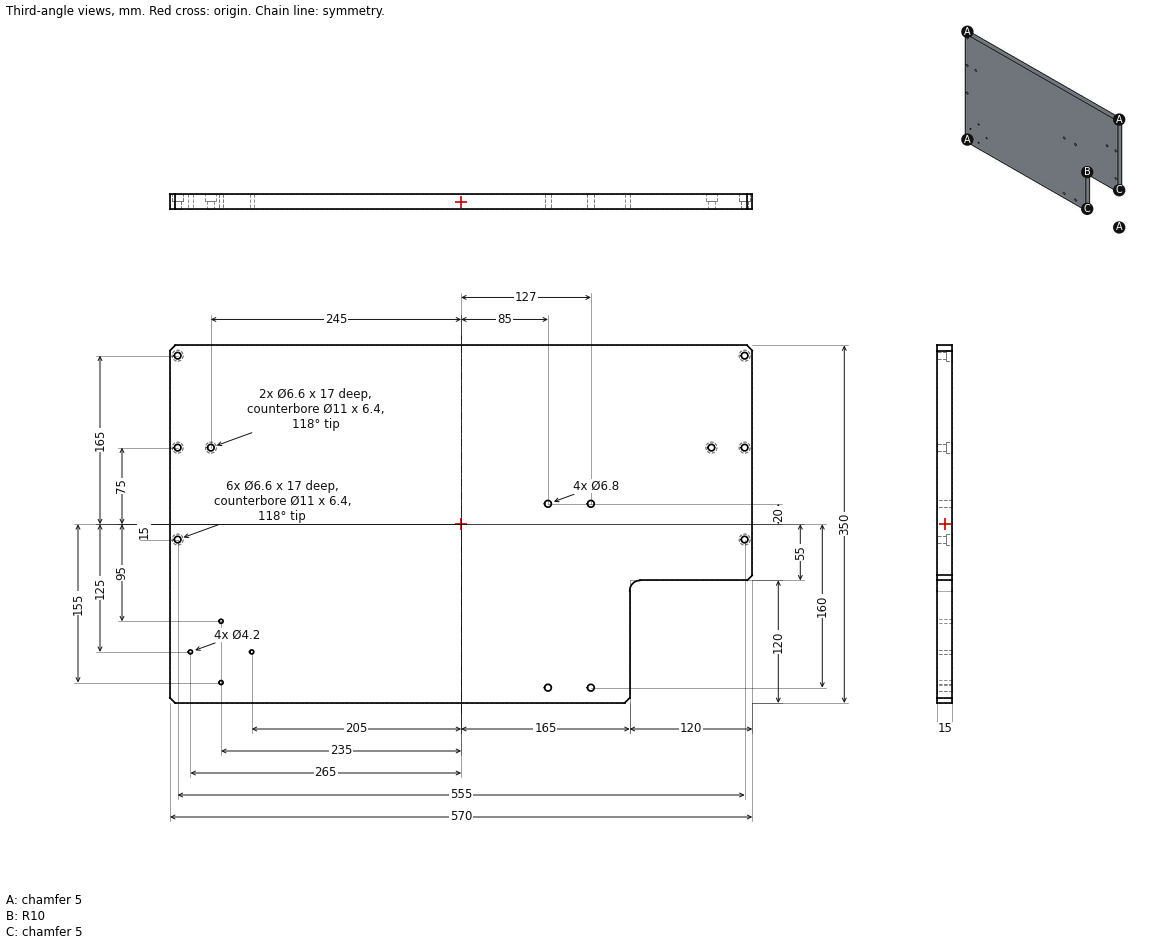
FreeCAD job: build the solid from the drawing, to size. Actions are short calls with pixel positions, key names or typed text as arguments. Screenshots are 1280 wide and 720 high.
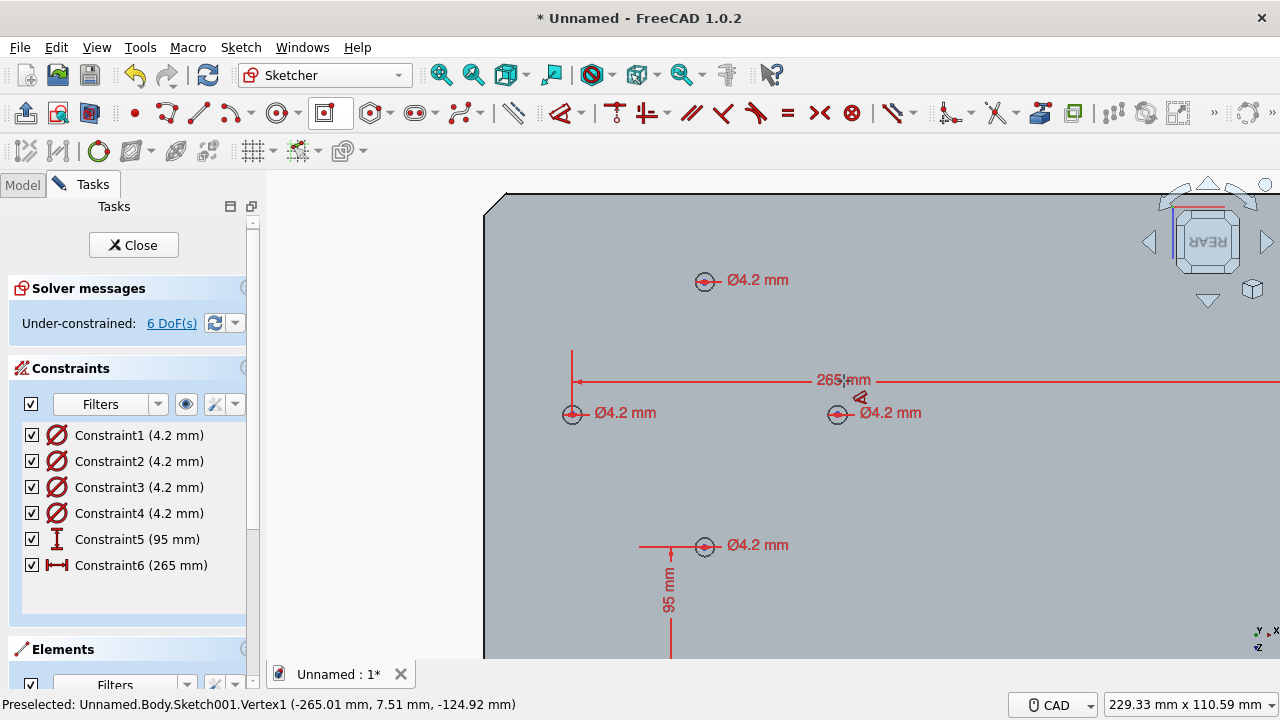
click(572, 415)
click(538, 523)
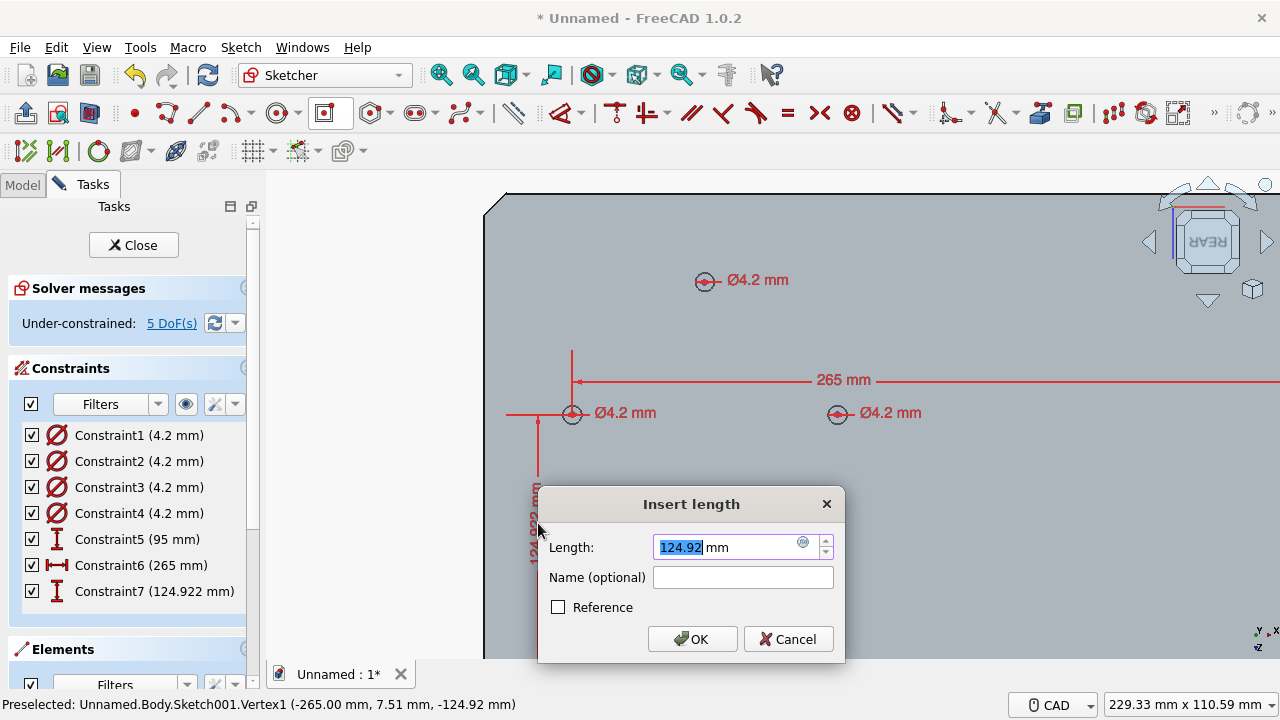
text(125)
key(Return)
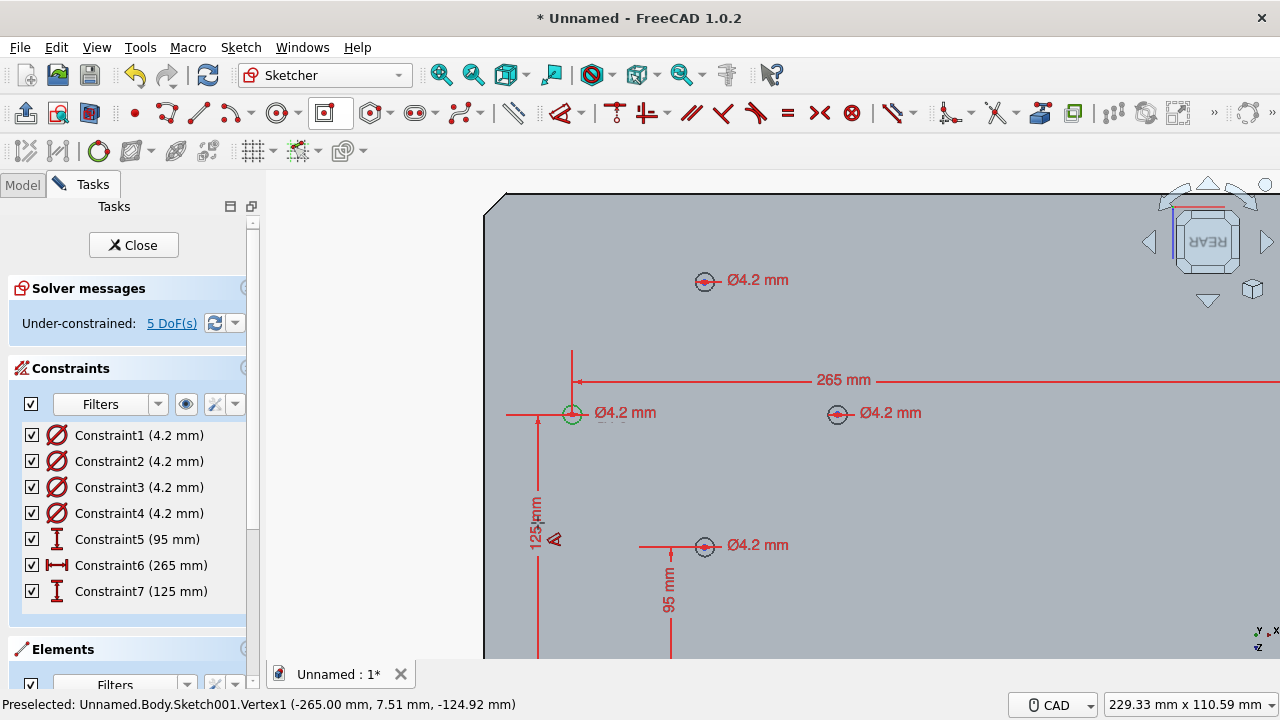
click(705, 547)
click(910, 513)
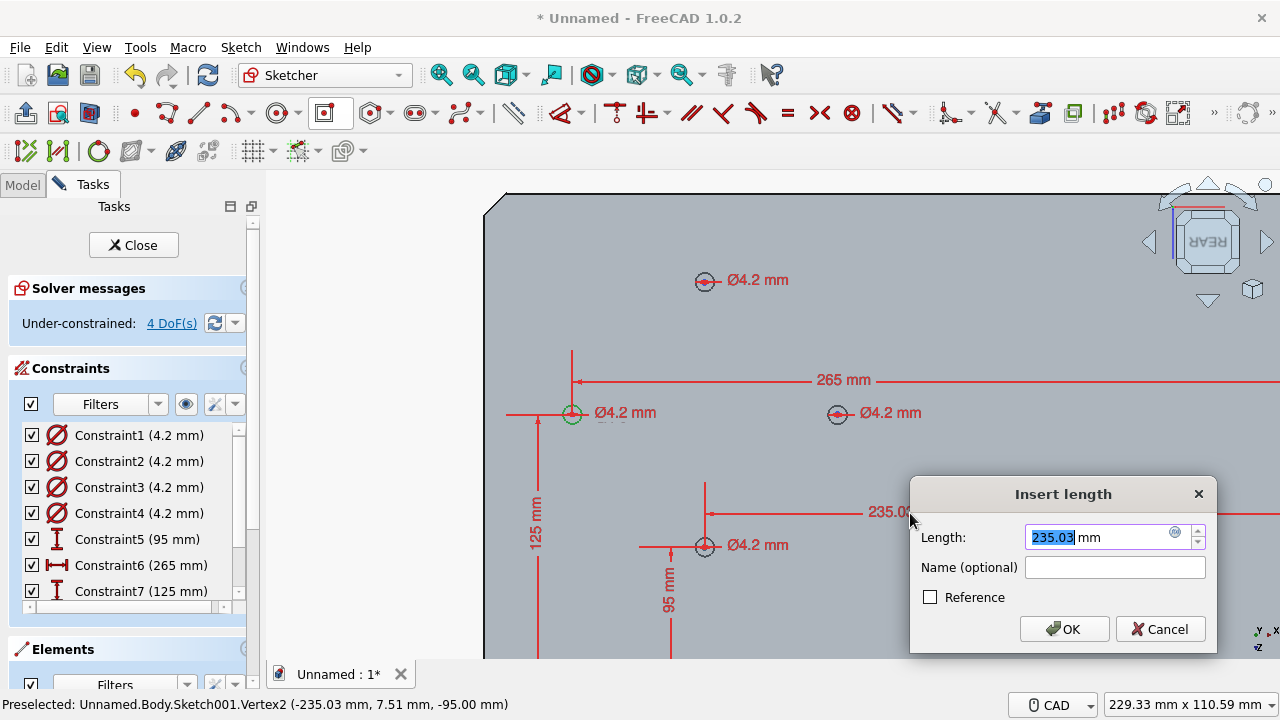
text(235)
key(Return)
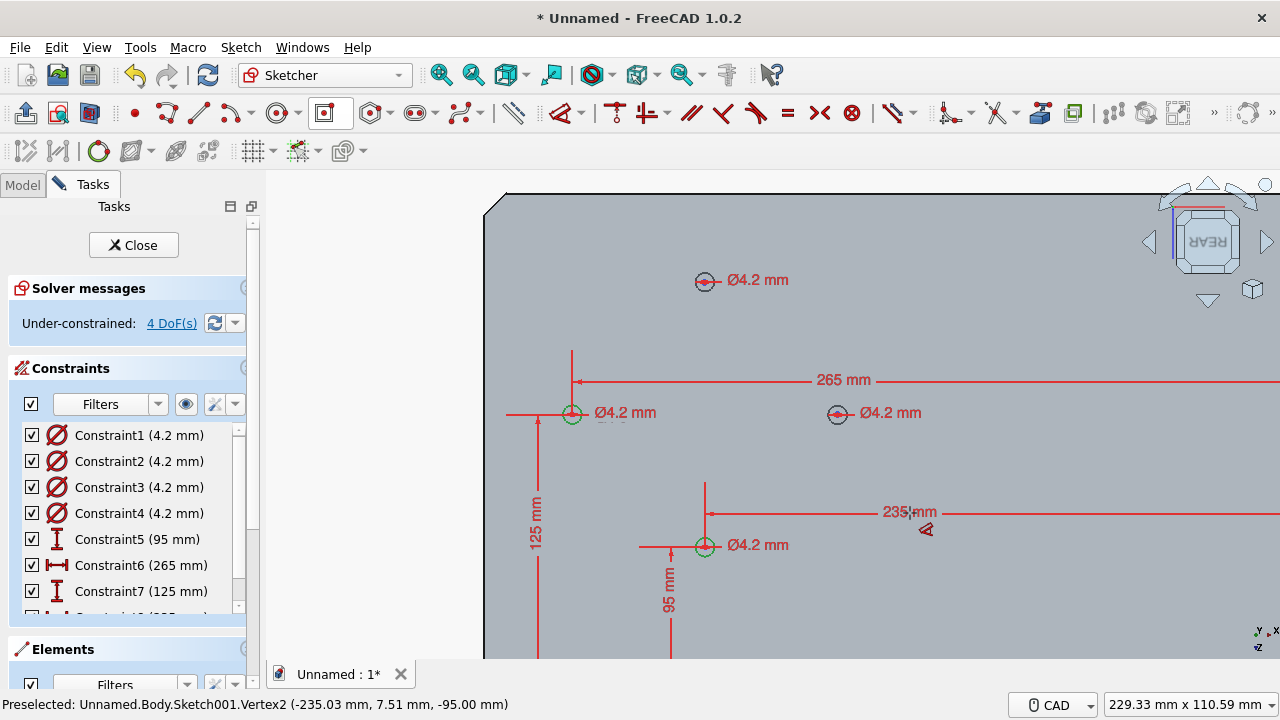
click(705, 282)
click(910, 248)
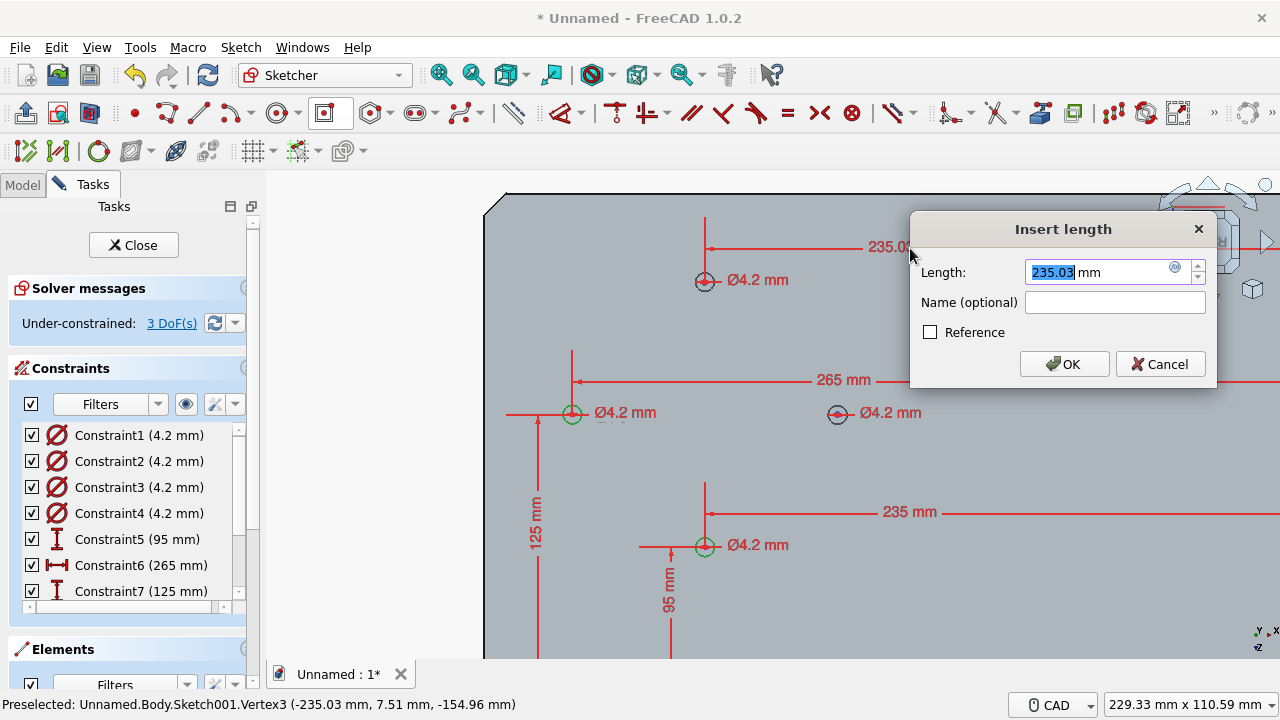
text(235)
key(Return)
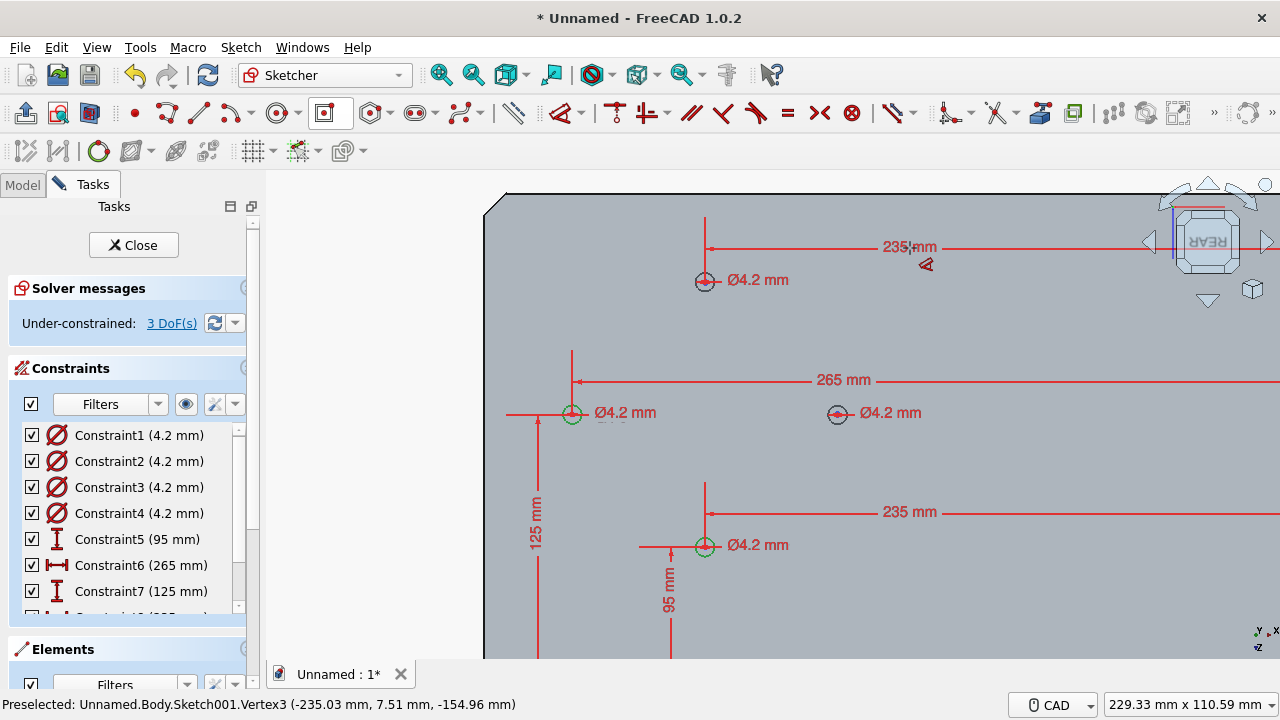
click(705, 282)
click(671, 457)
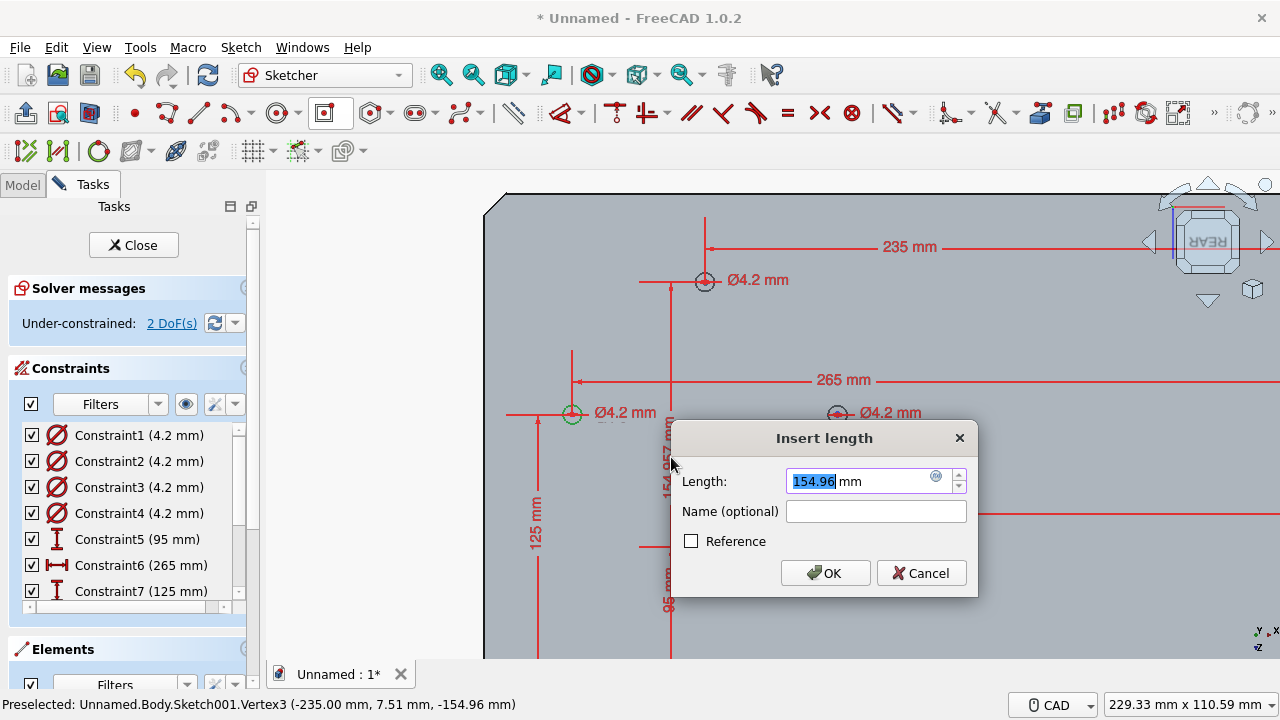
text(155)
key(Return)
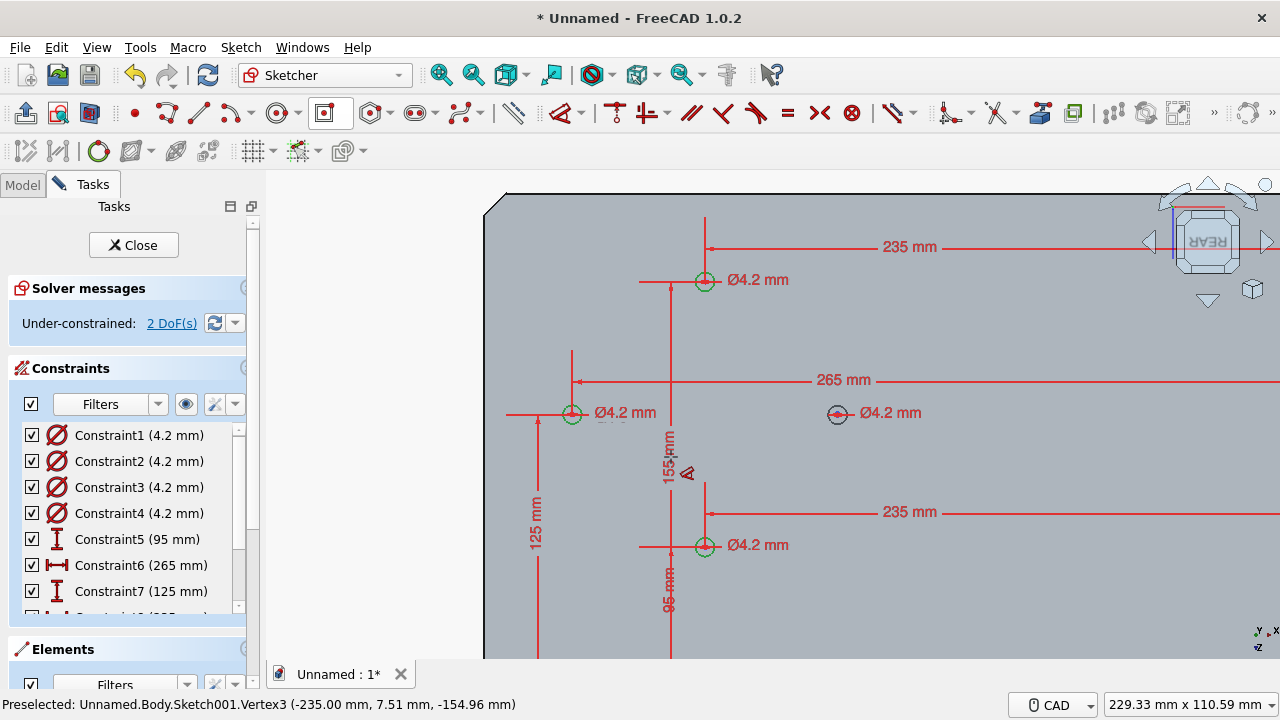
click(838, 415)
click(976, 381)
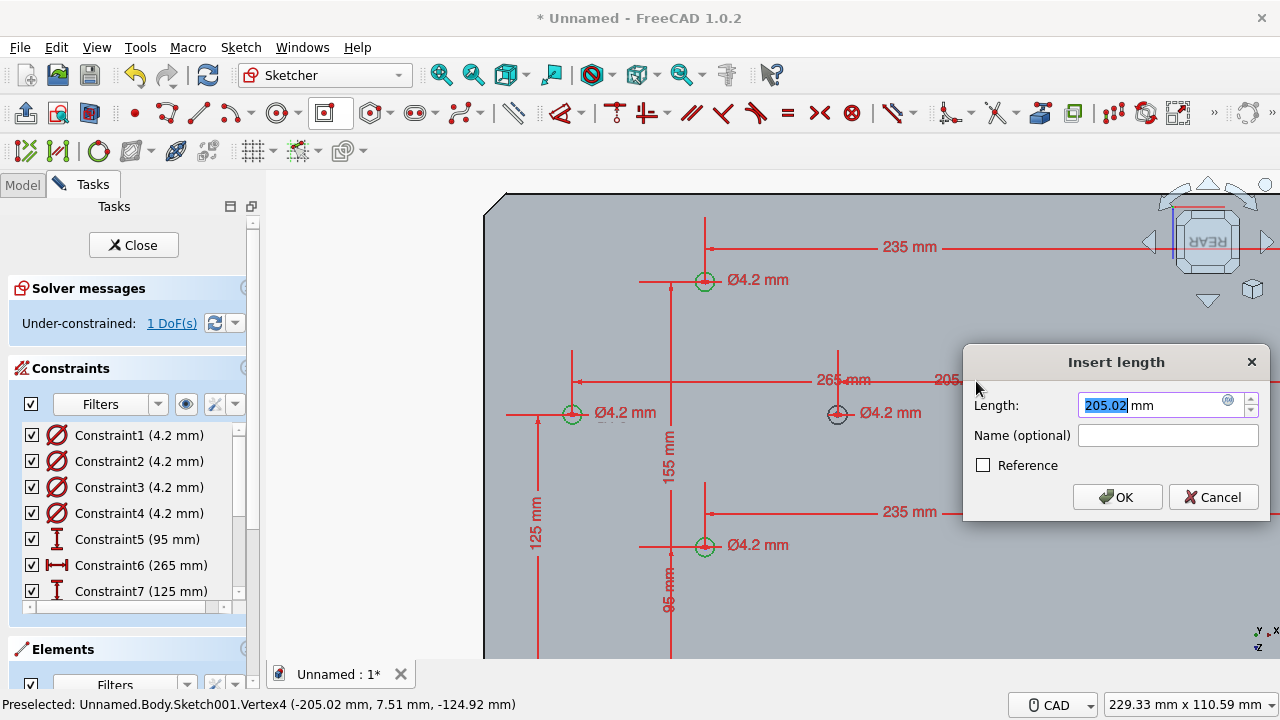
text(205)
key(Return)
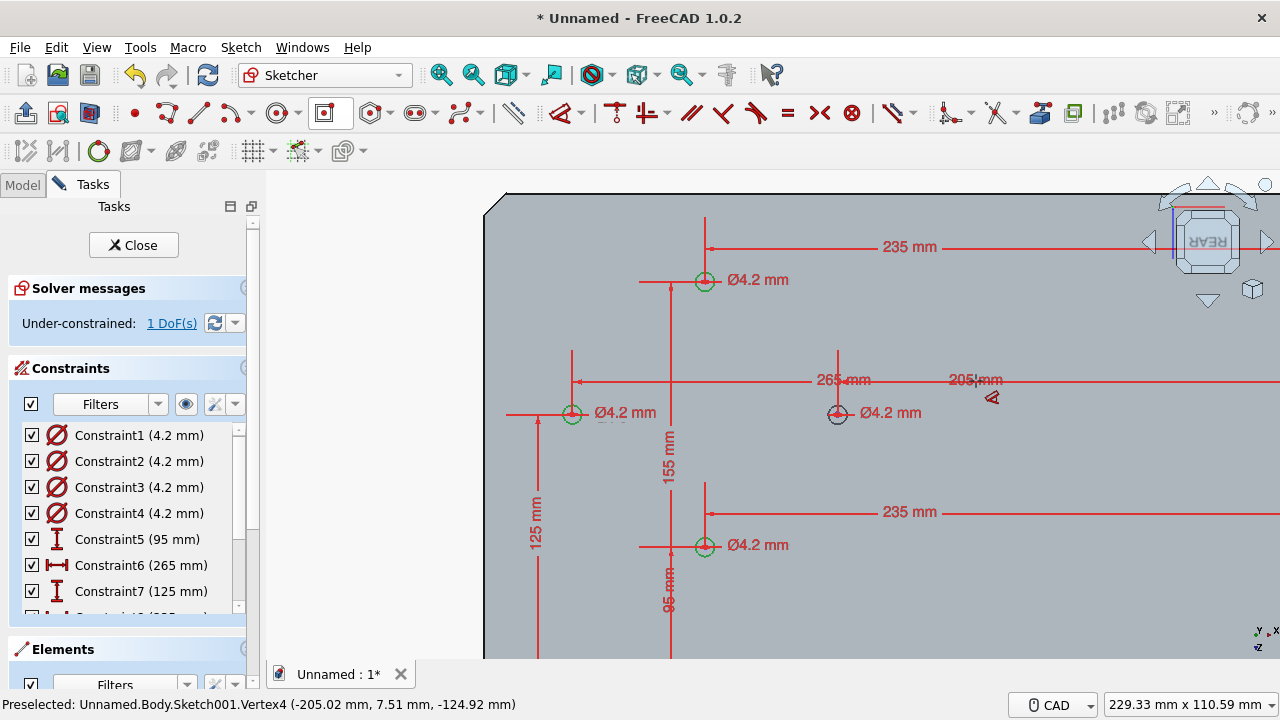
click(838, 415)
click(804, 523)